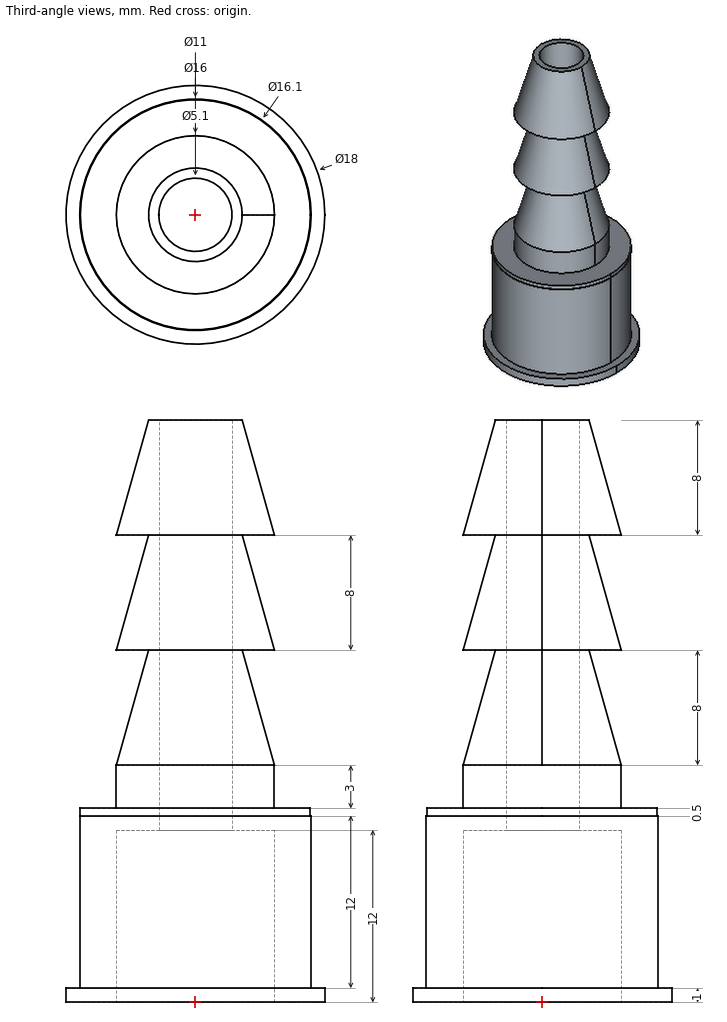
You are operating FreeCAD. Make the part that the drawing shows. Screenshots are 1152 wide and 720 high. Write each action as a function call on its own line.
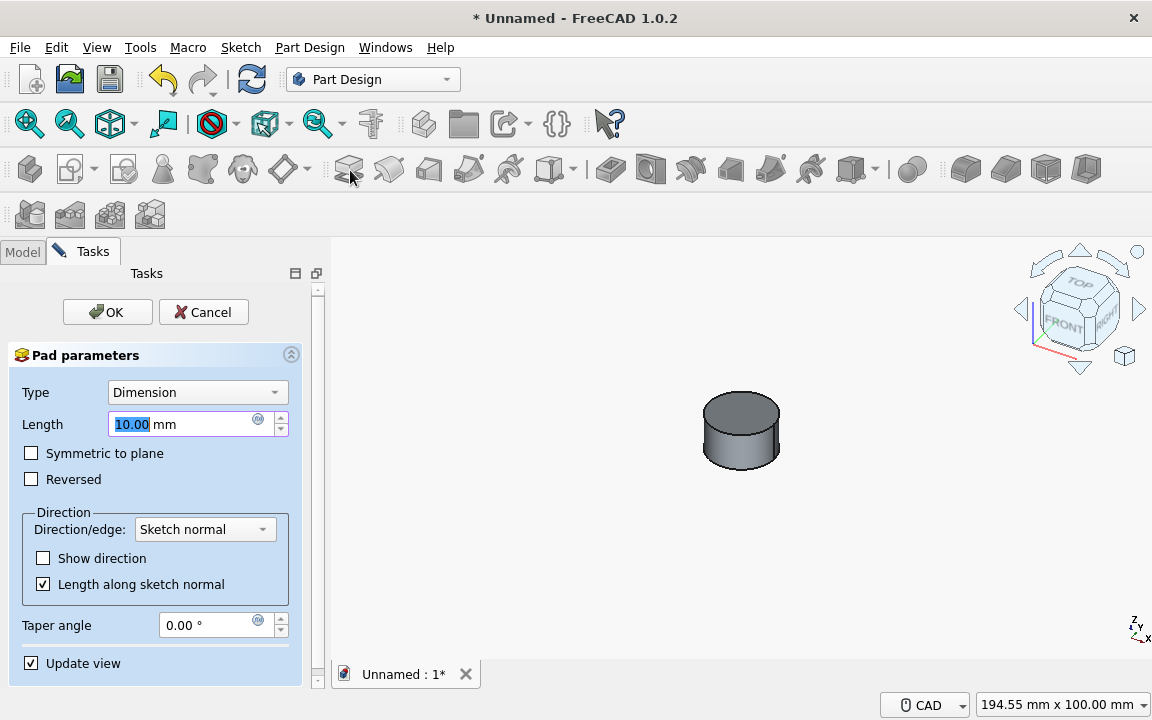
text(1)
key(Tab)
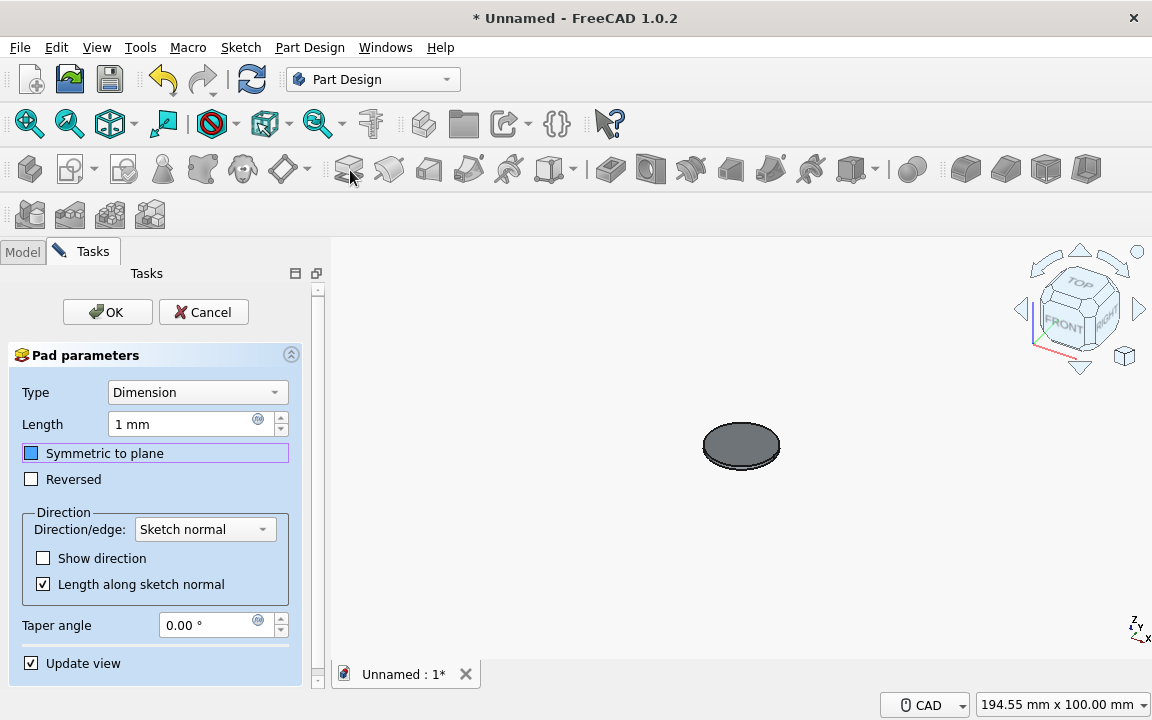
click(108, 312)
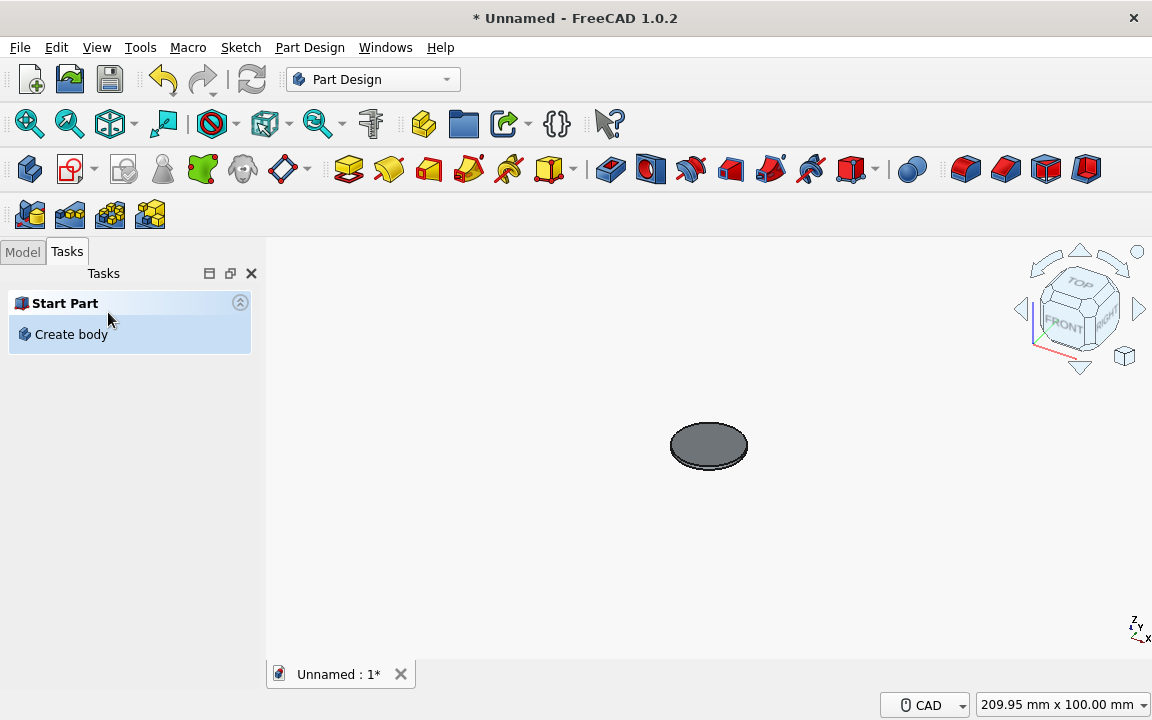
key(v)
key(f)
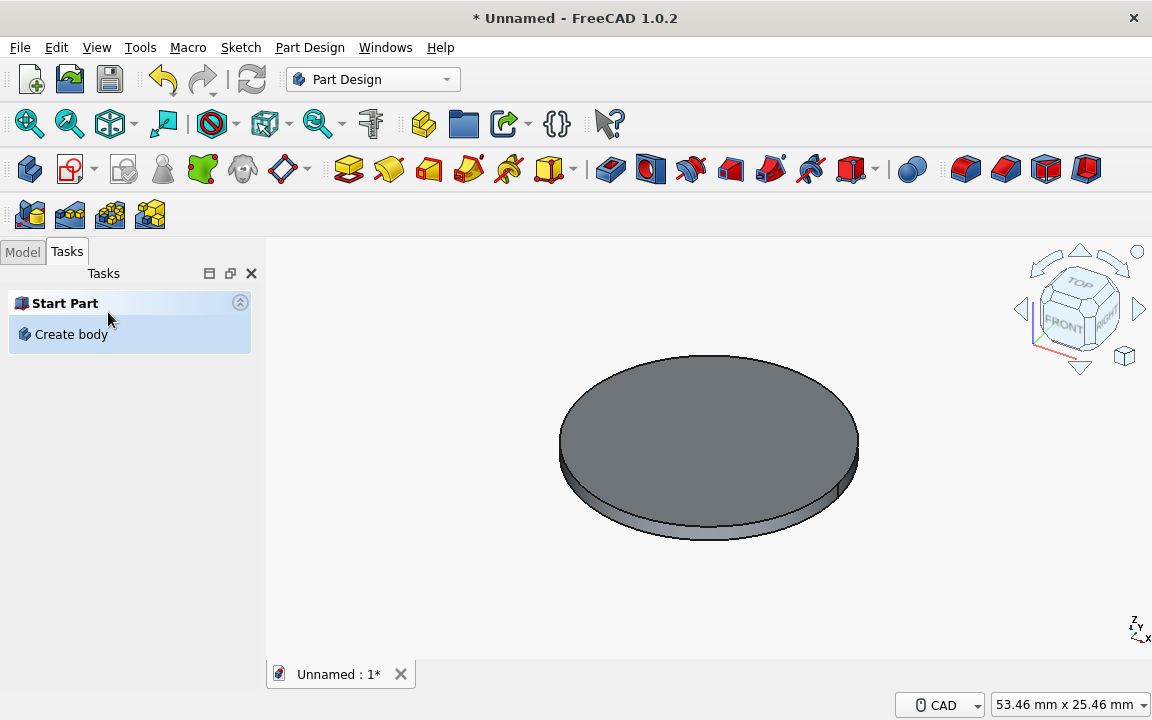
click(709, 440)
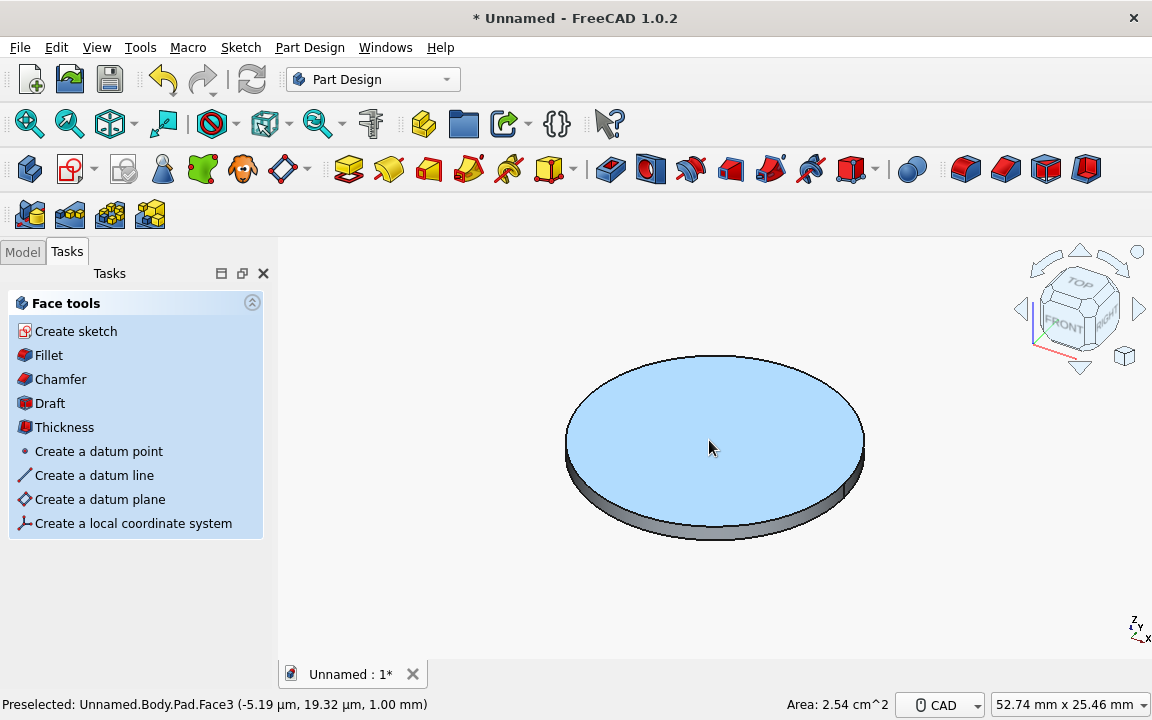
click(70, 170)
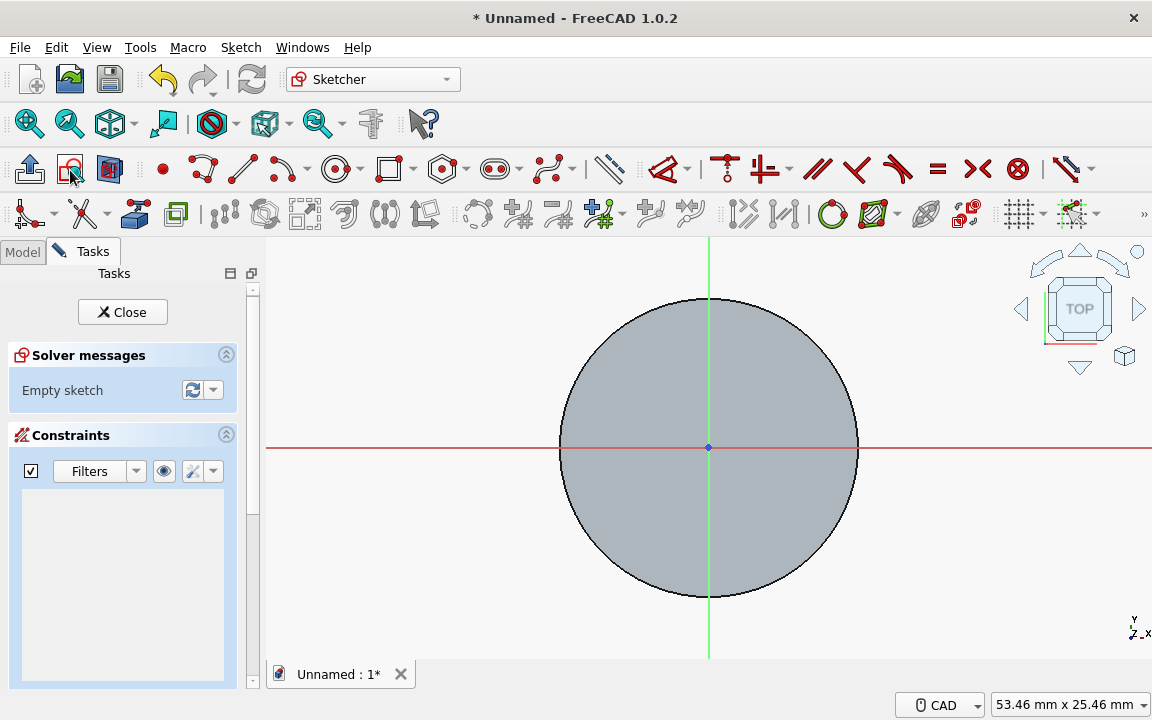
key(g)
key(c)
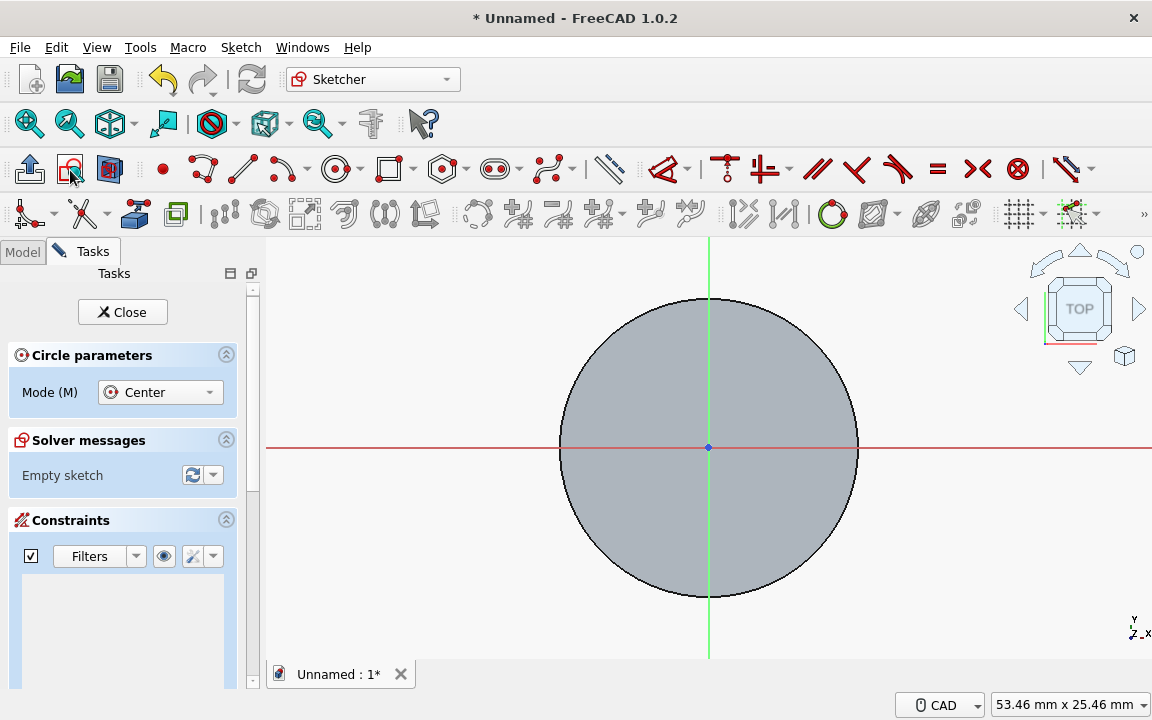
click(709, 448)
click(803, 354)
key(Escape)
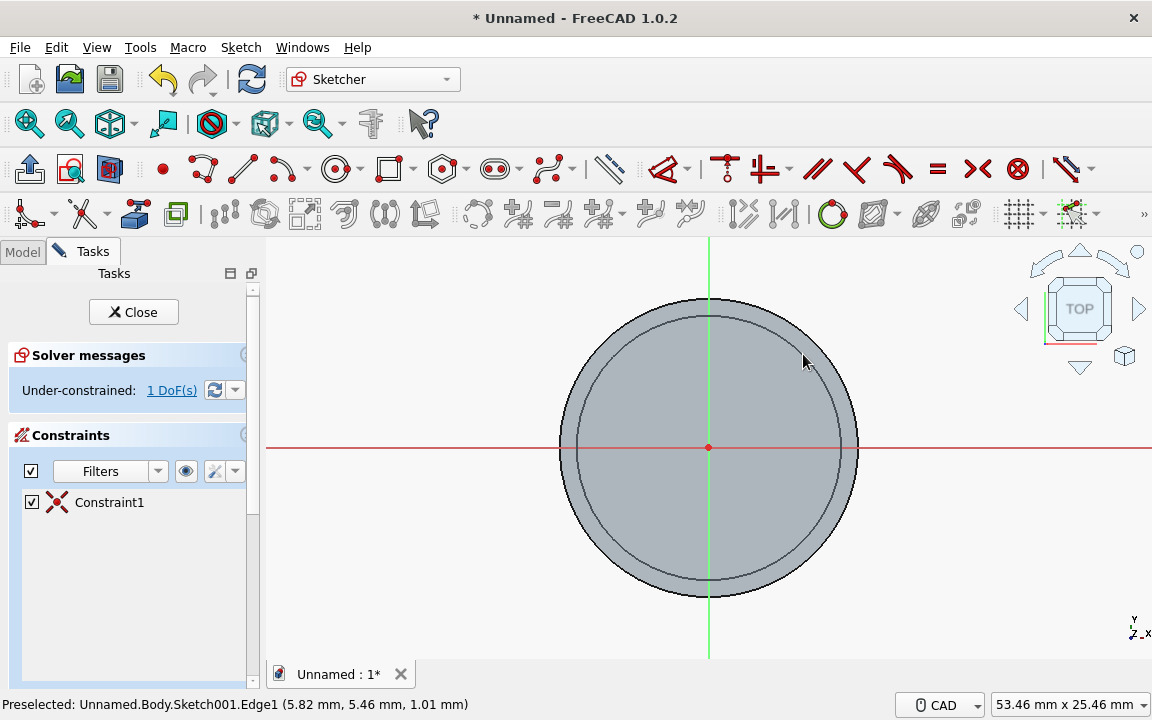
key(d)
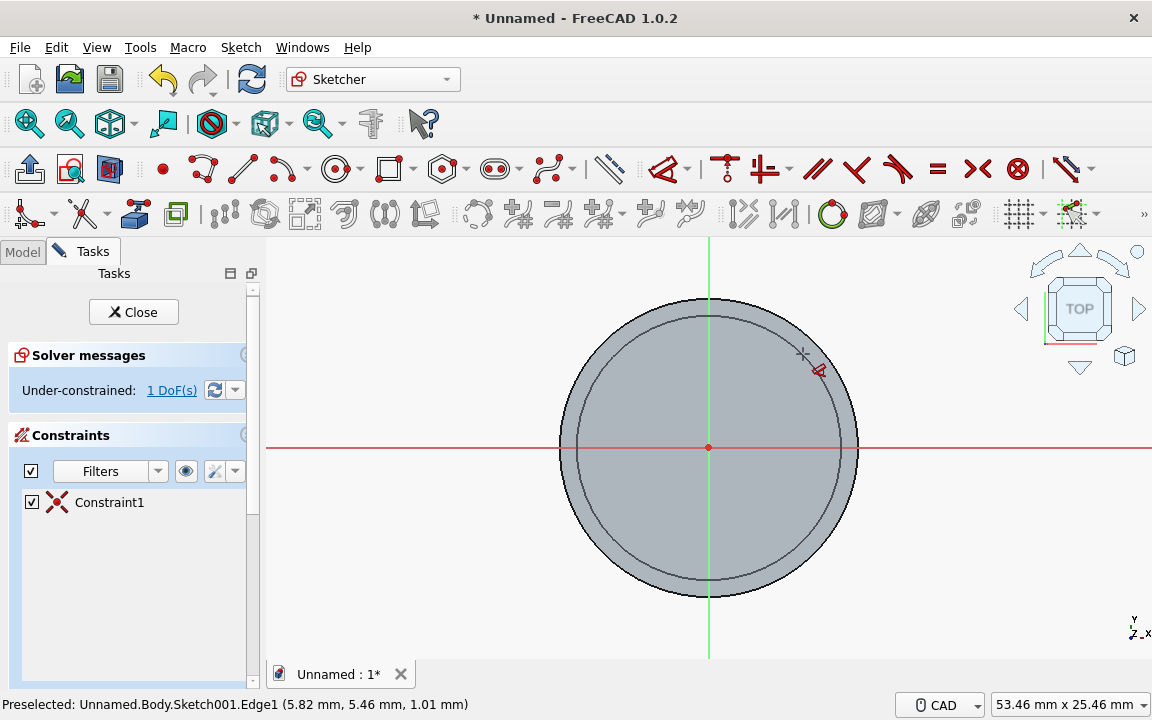
click(802, 354)
click(825, 331)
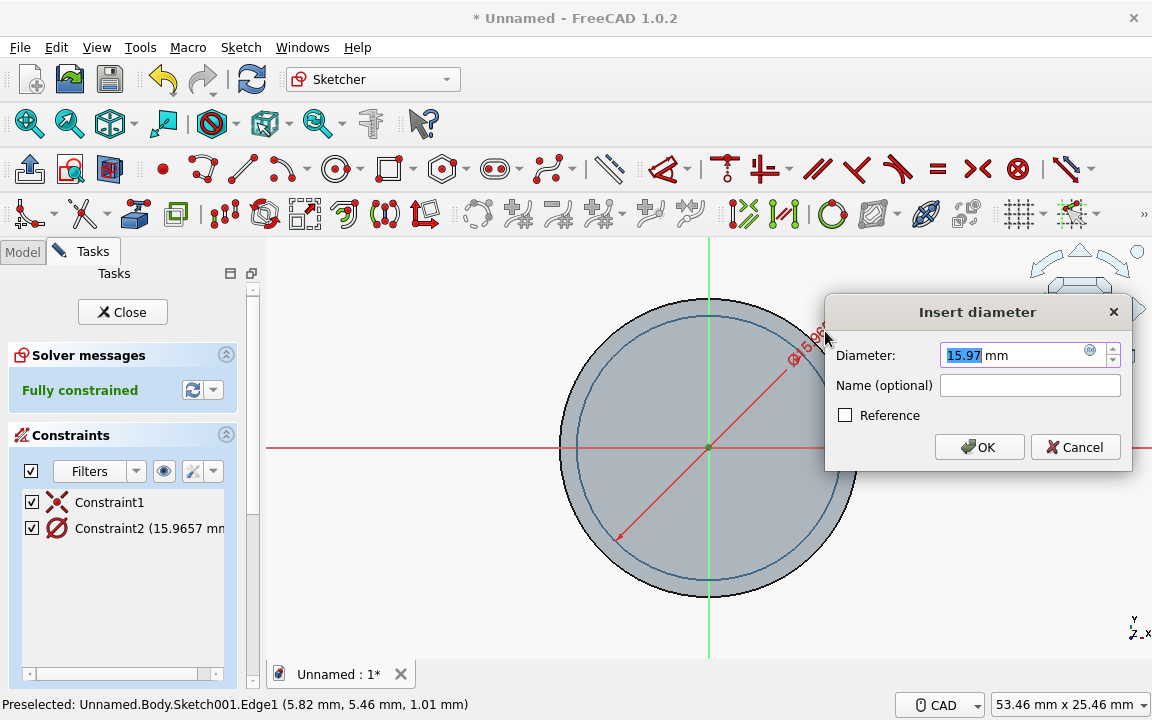
text(16.1)
key(Return)
key(Escape)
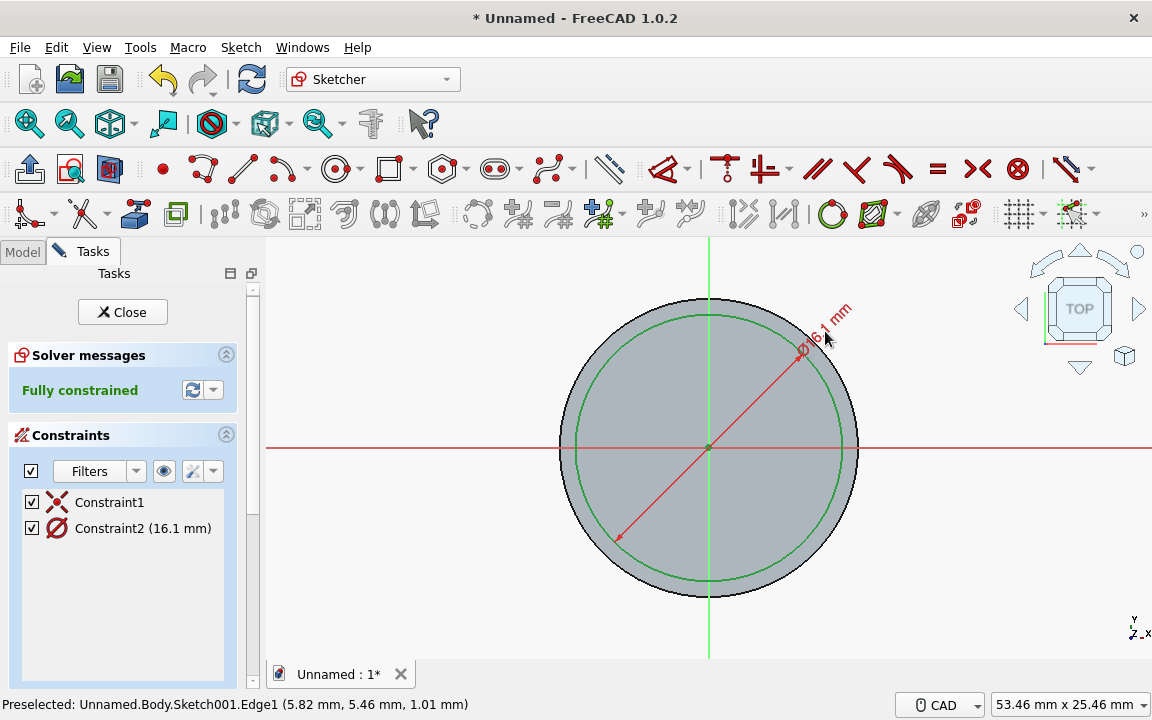
click(123, 312)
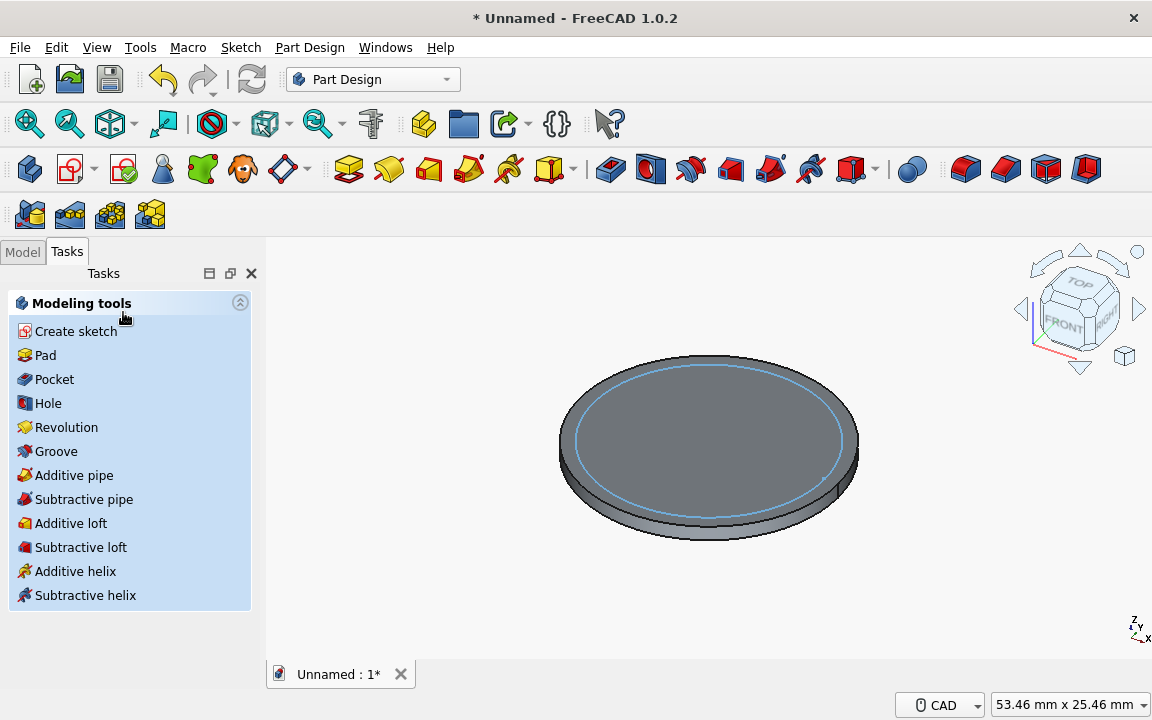
click(350, 170)